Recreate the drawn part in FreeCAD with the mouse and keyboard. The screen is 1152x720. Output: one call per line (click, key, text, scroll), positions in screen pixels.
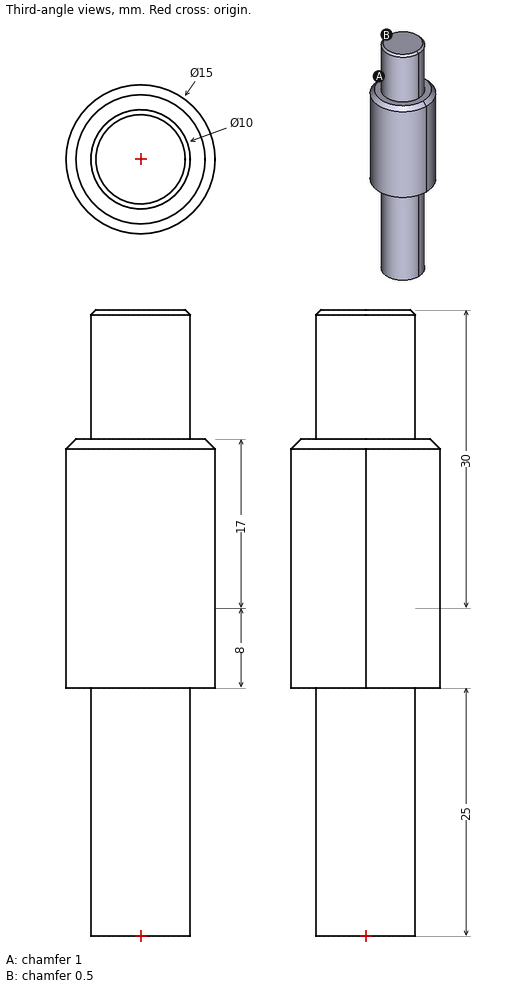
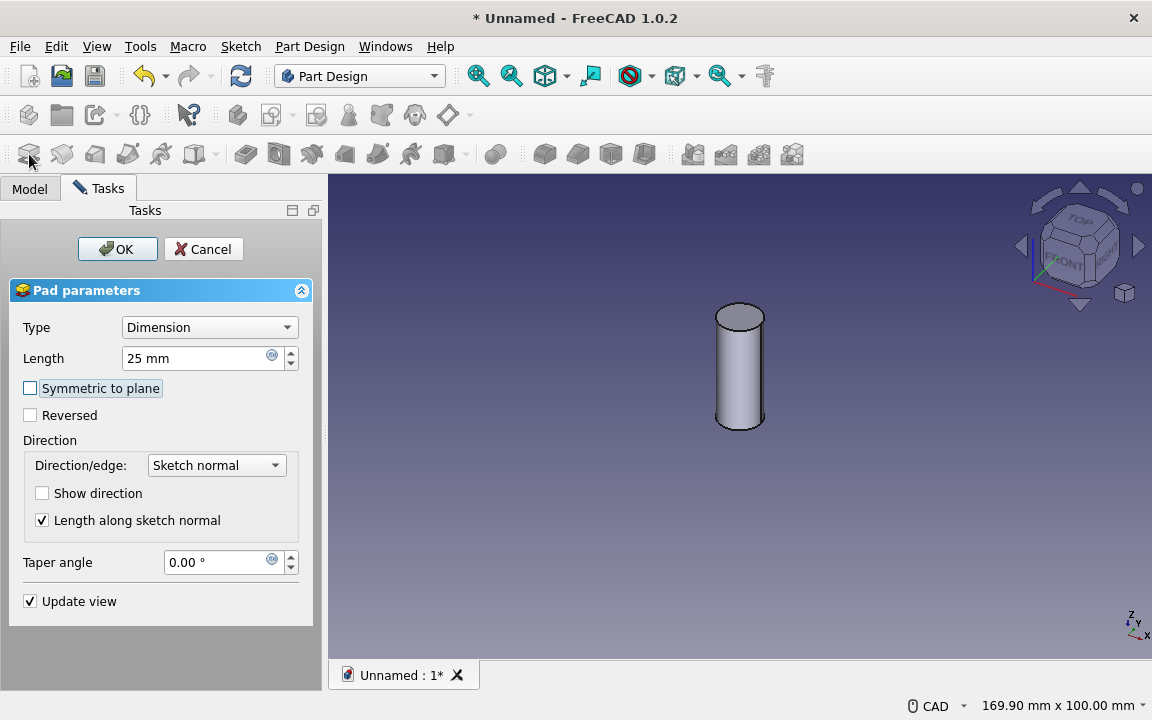
click(118, 249)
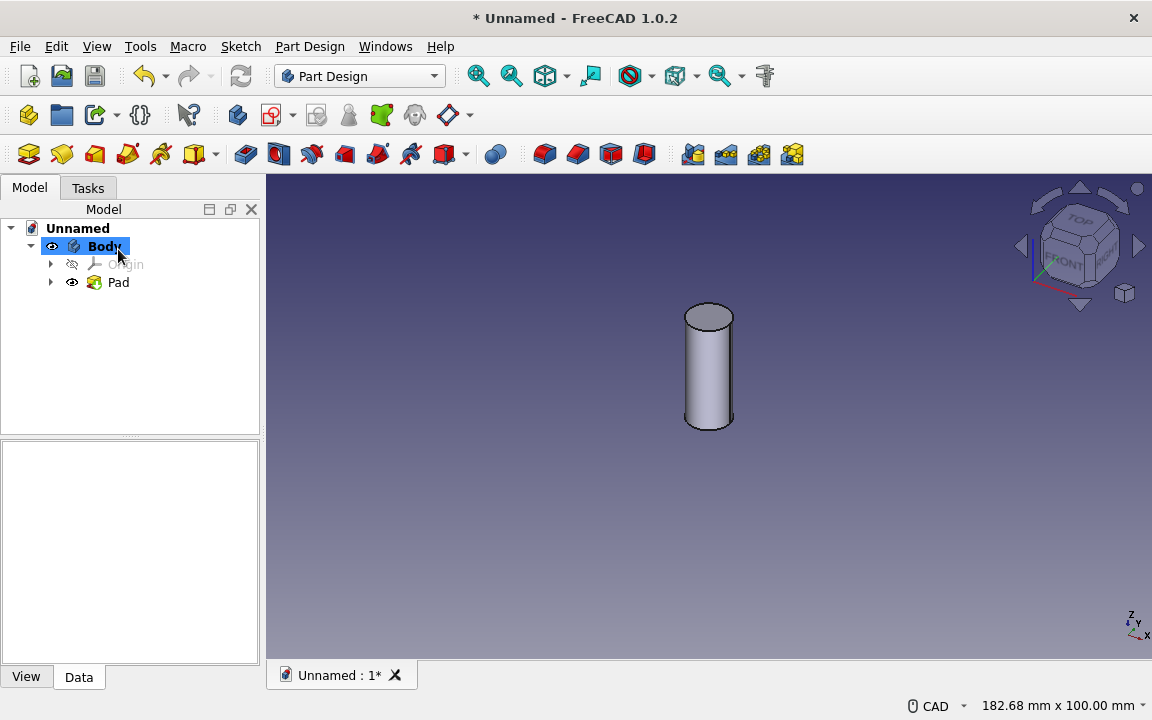
click(479, 76)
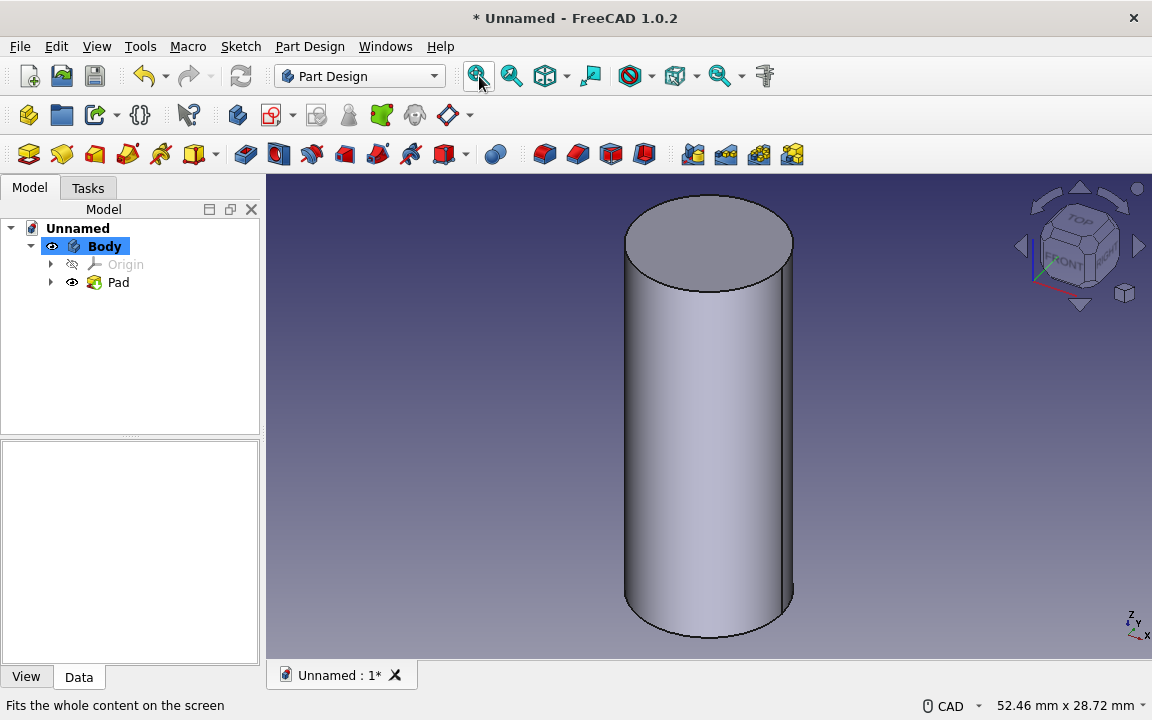
click(709, 243)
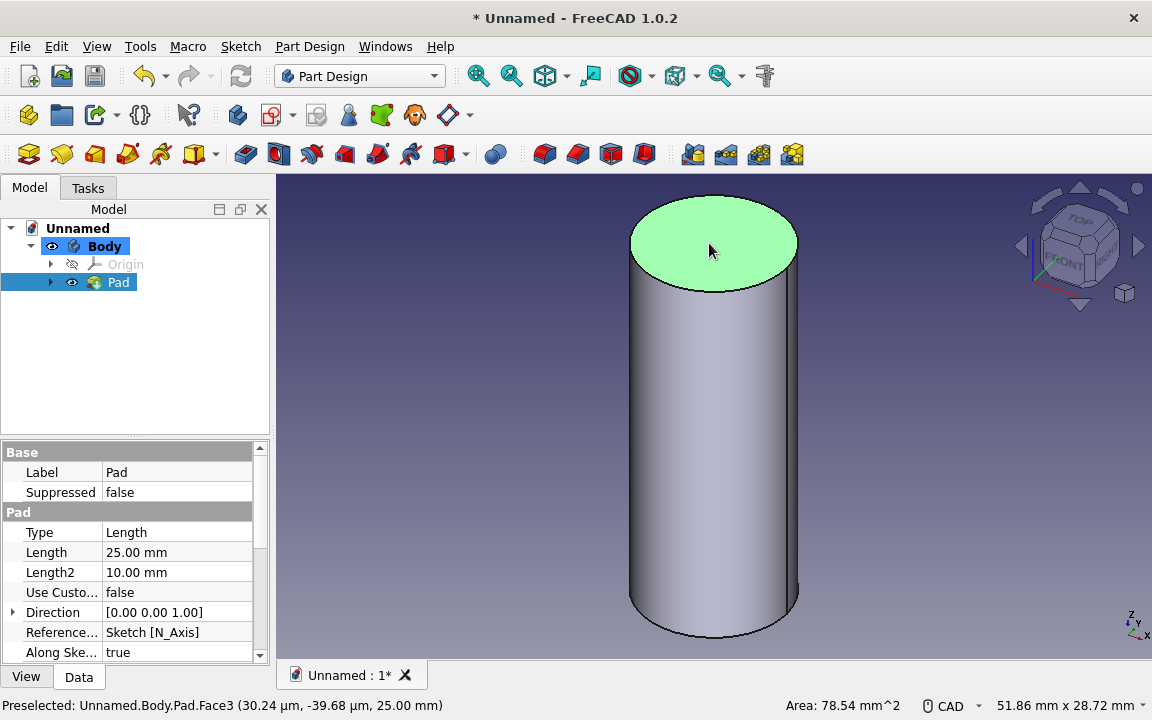
click(270, 116)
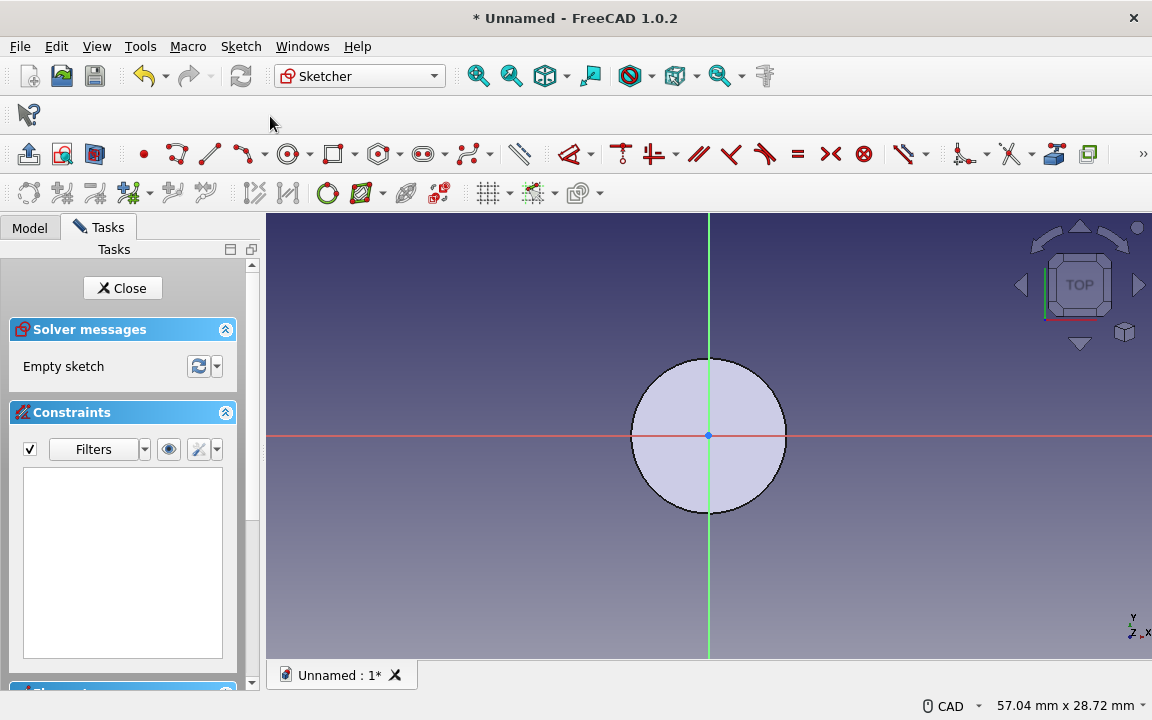
key(g)
key(c)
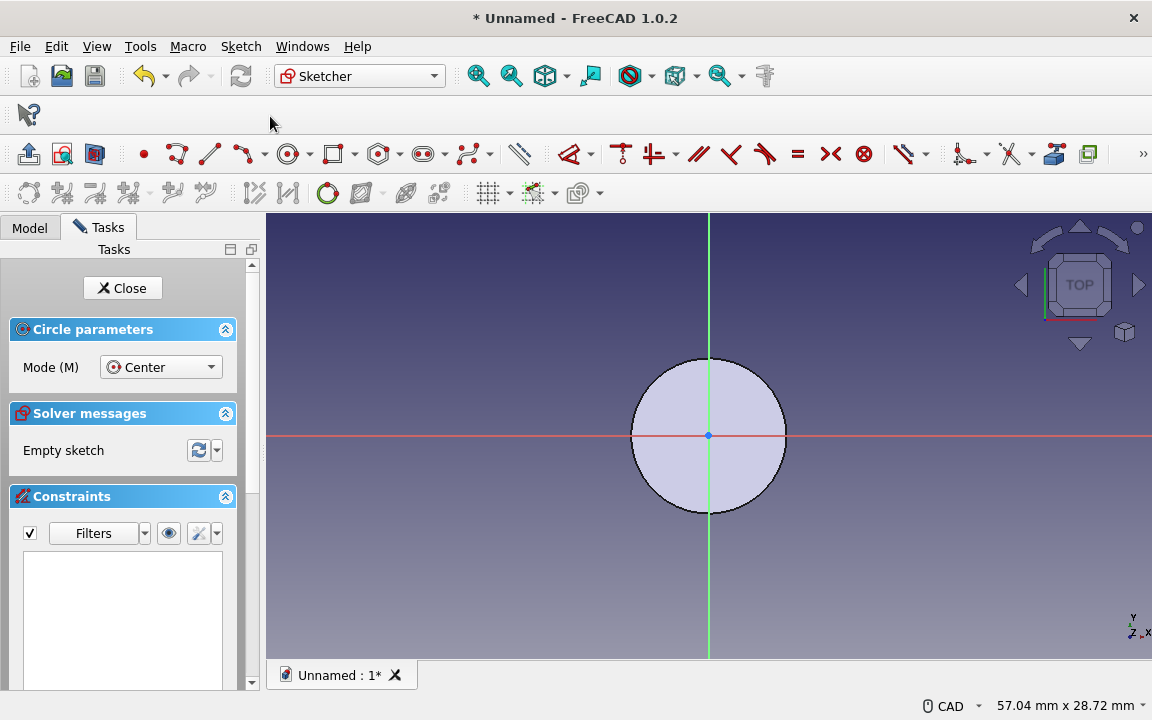
click(709, 436)
click(791, 354)
key(Escape)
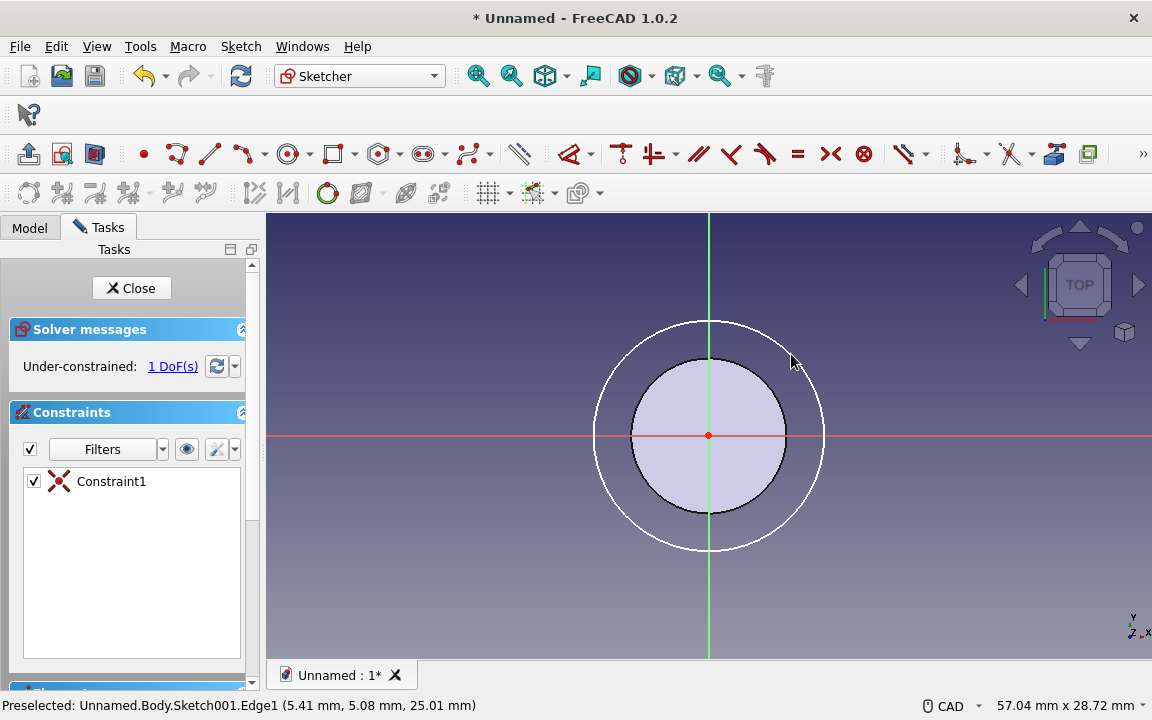
key(d)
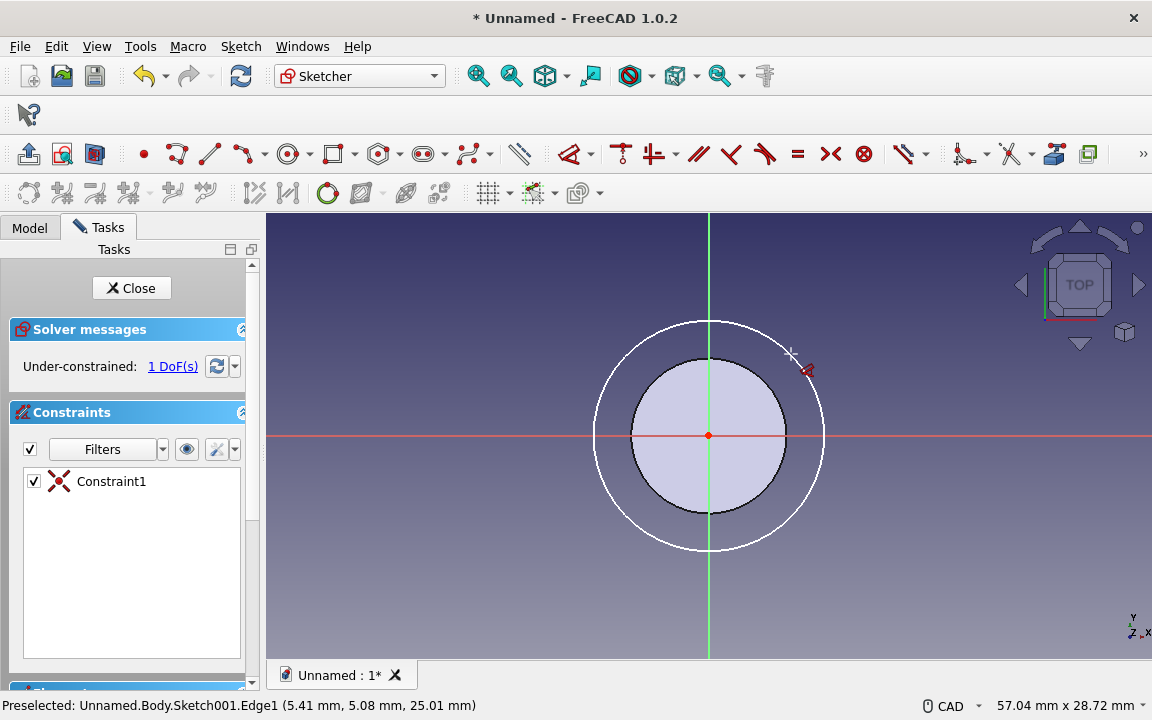
click(790, 354)
click(813, 331)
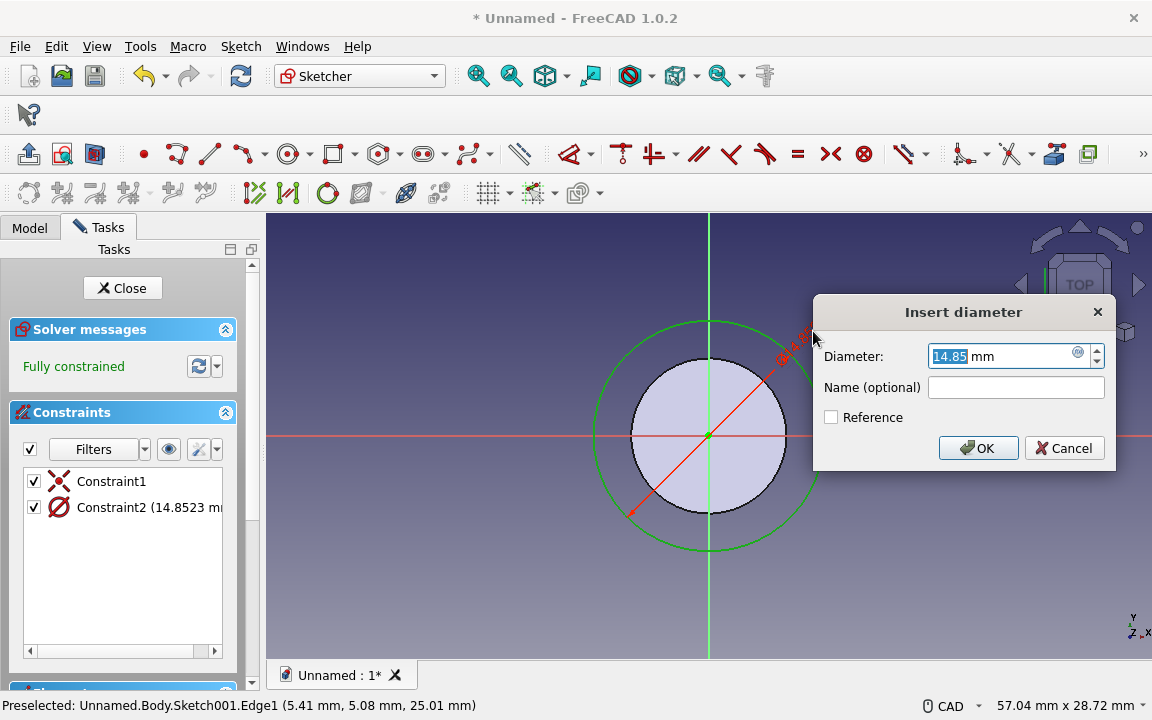
text(15)
key(Return)
key(Escape)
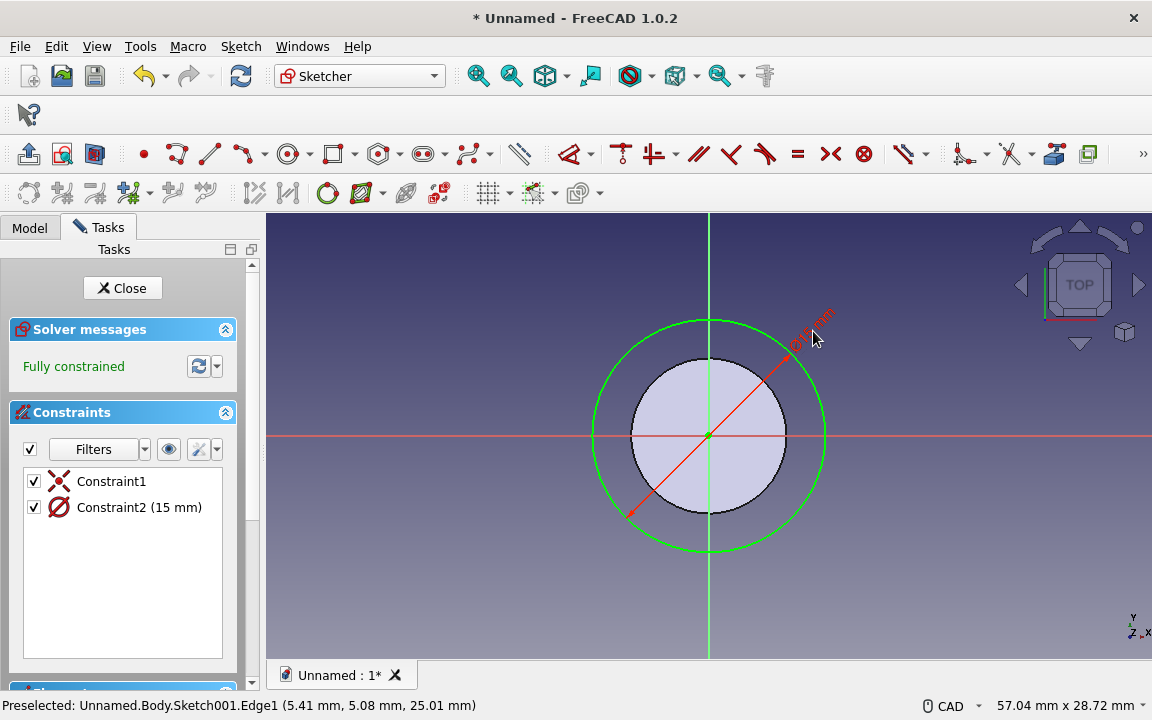
click(123, 288)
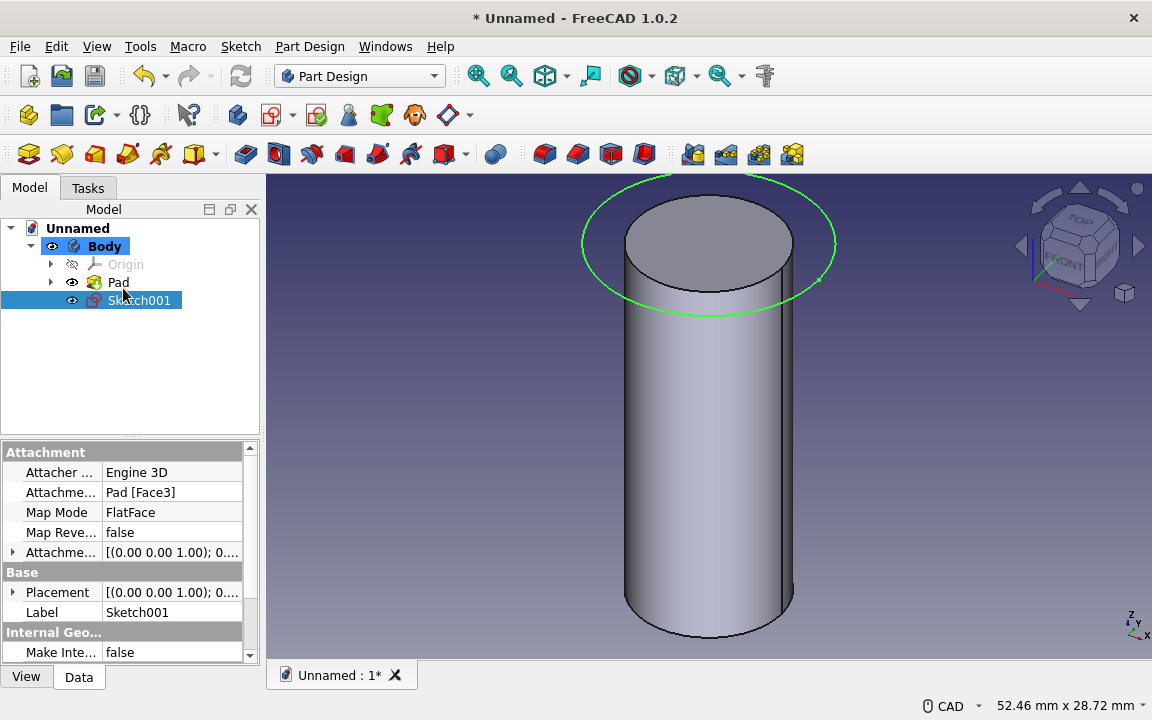
click(29, 154)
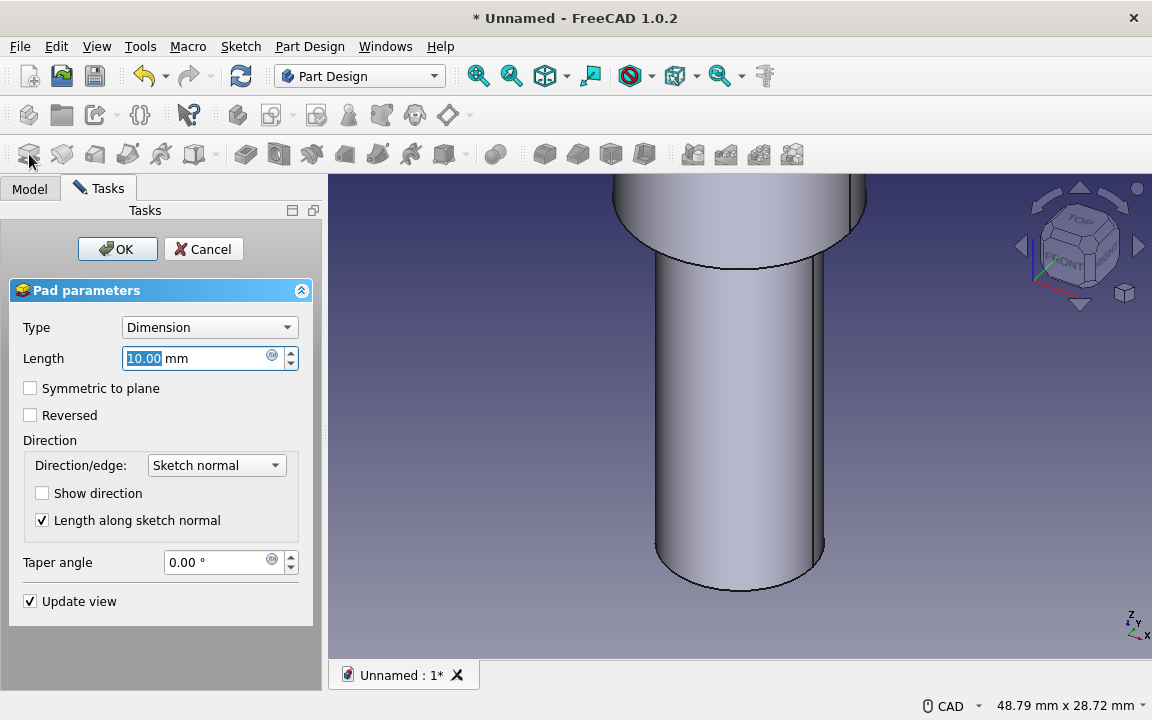
text(8)
key(Tab)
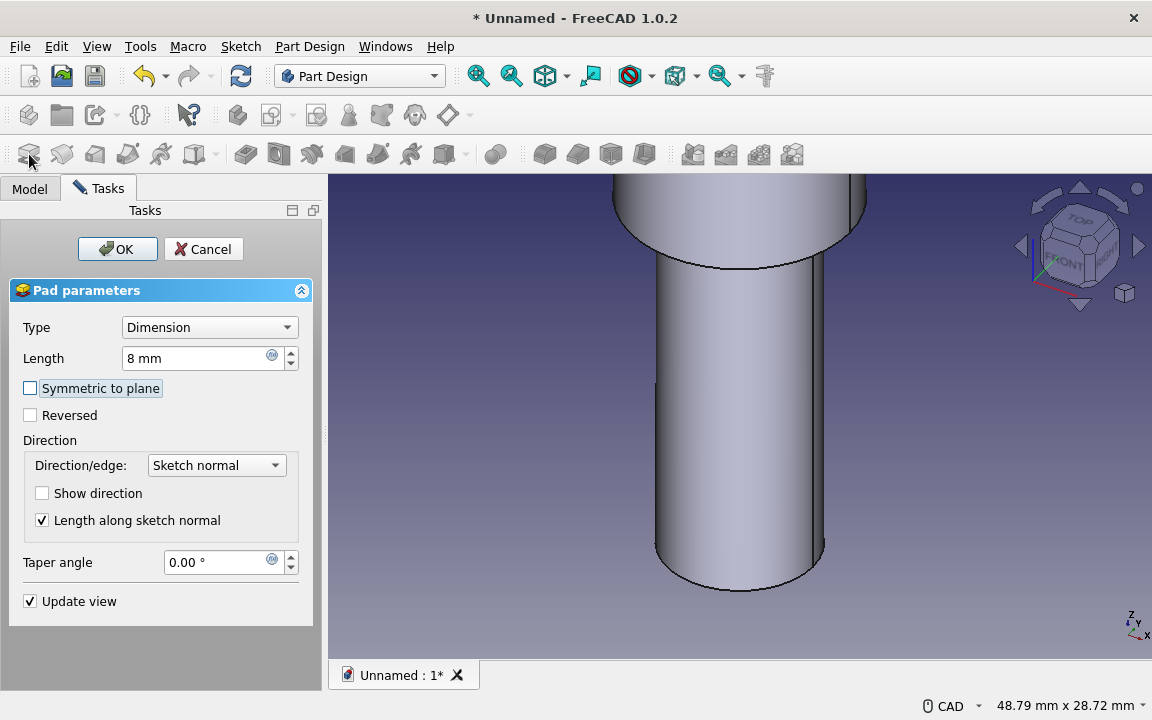
click(118, 249)